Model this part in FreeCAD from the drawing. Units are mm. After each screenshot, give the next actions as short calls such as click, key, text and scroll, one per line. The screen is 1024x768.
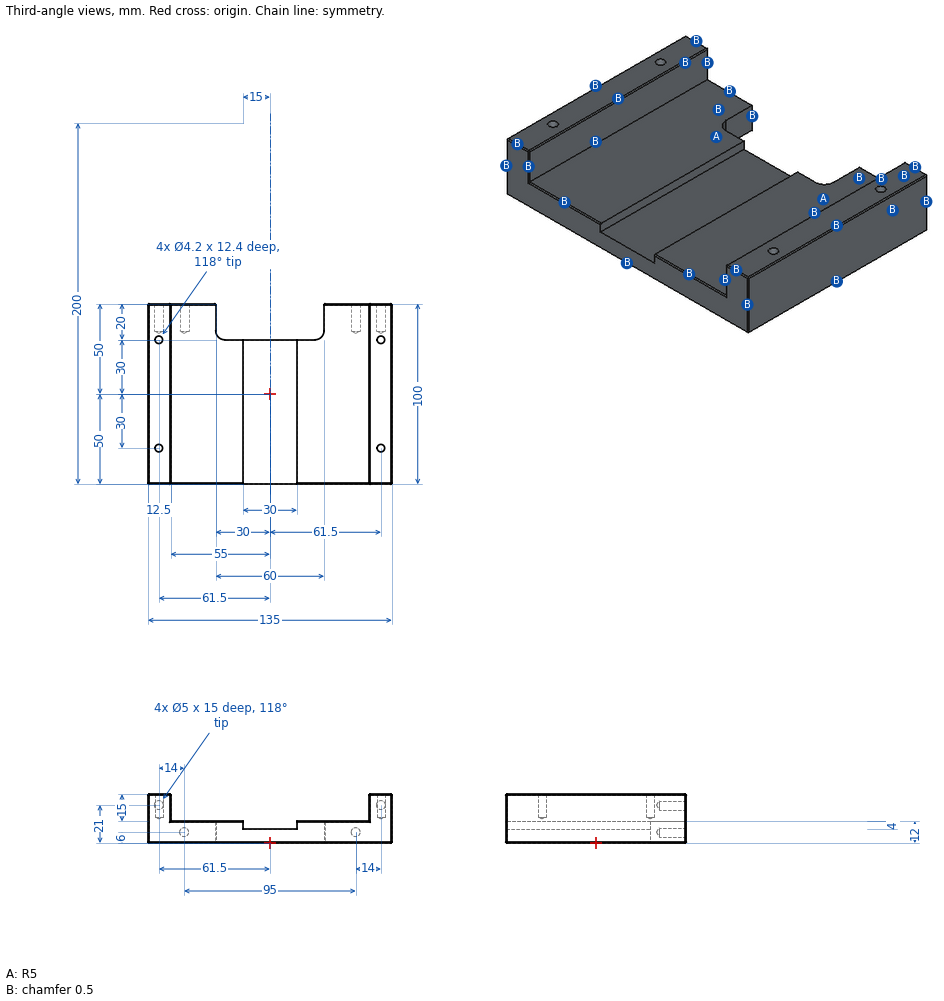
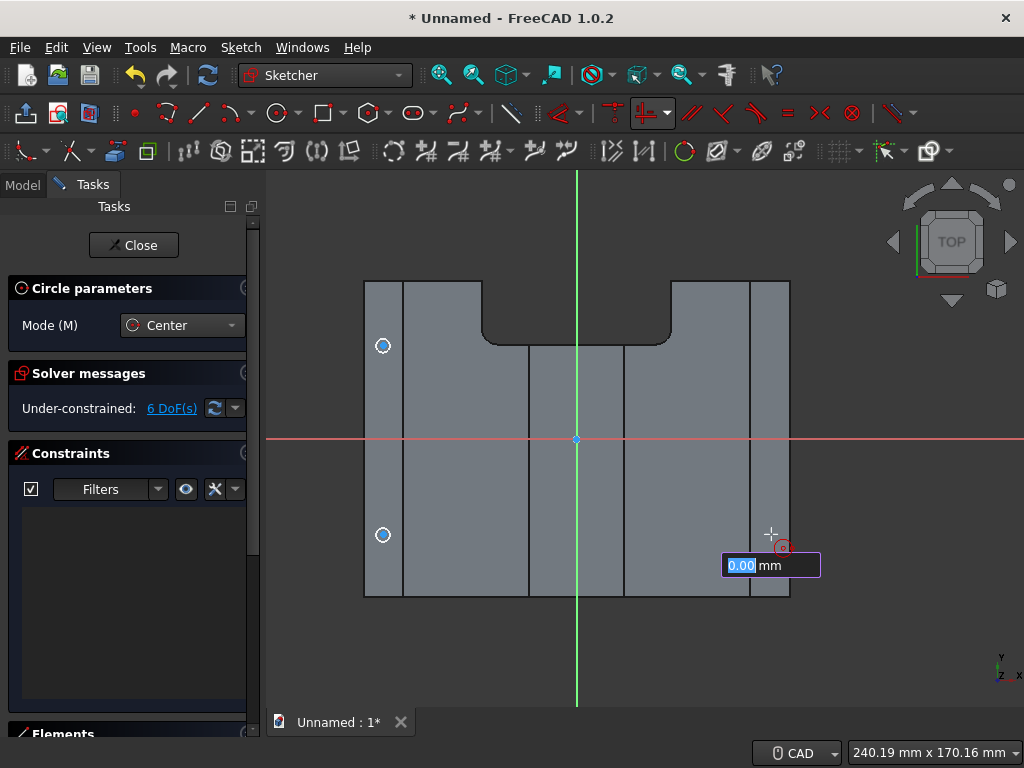
scroll(775, 529, up, 5)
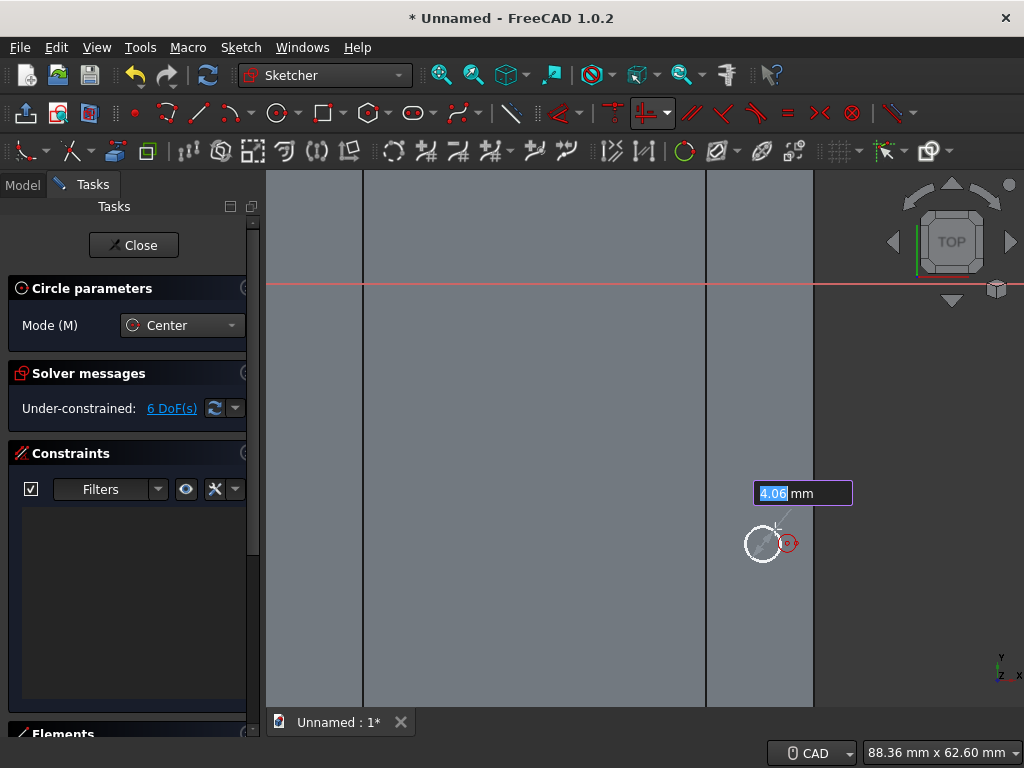
click(775, 528)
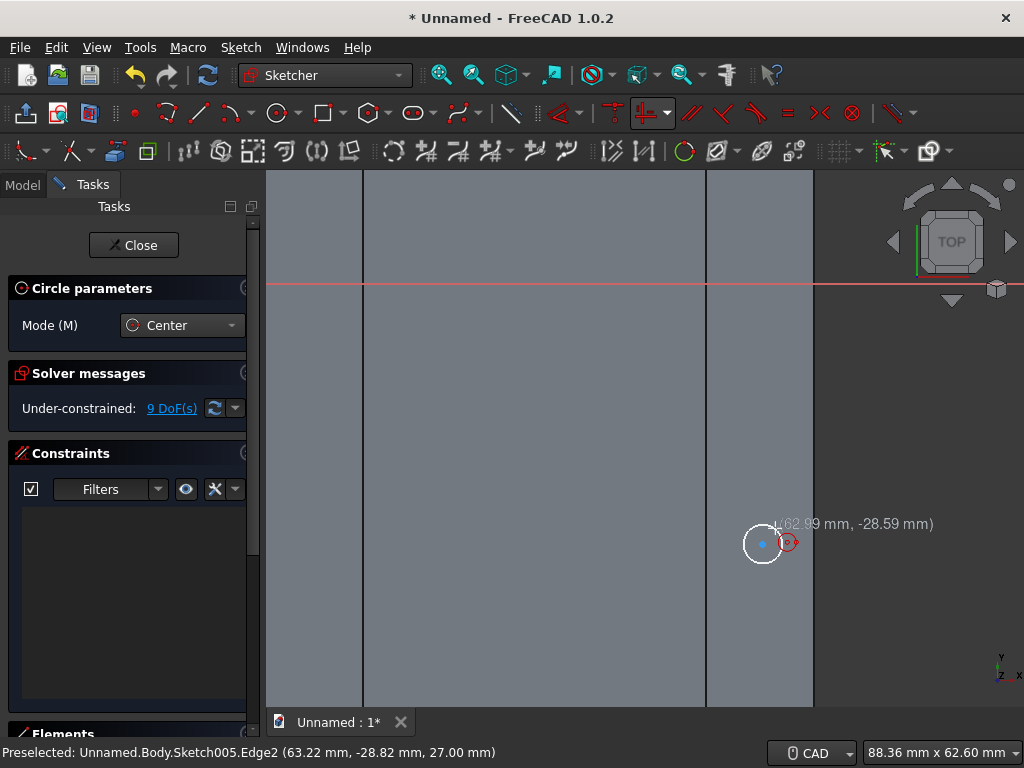
scroll(775, 529, down, 5)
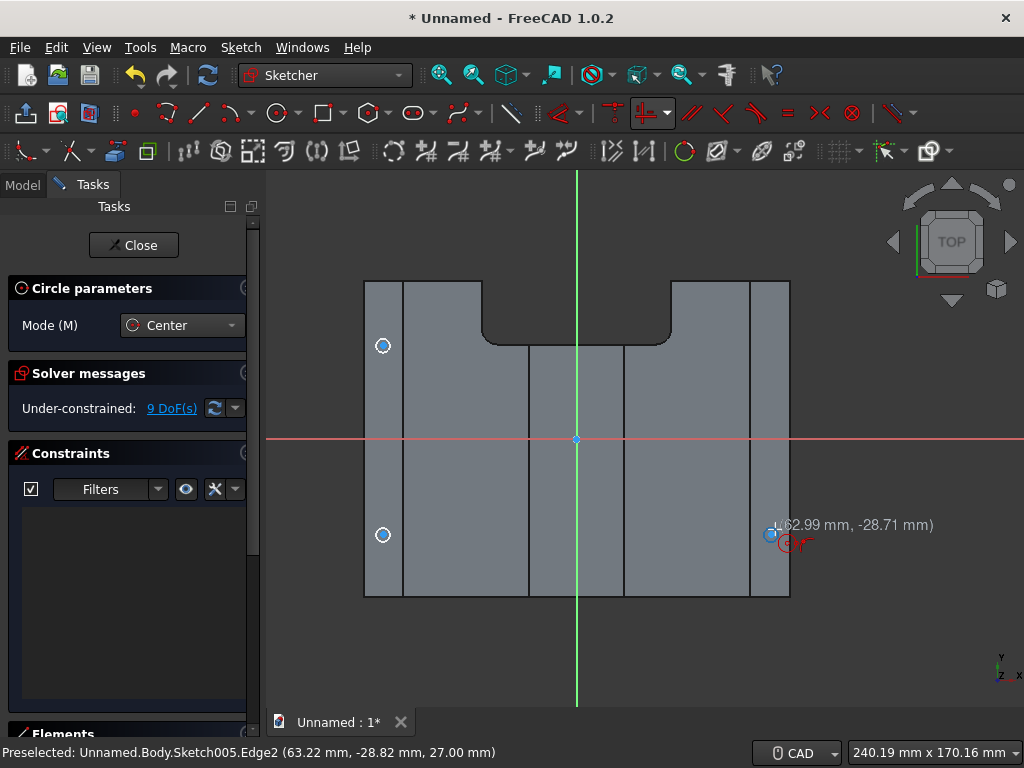
scroll(771, 345, up, 7)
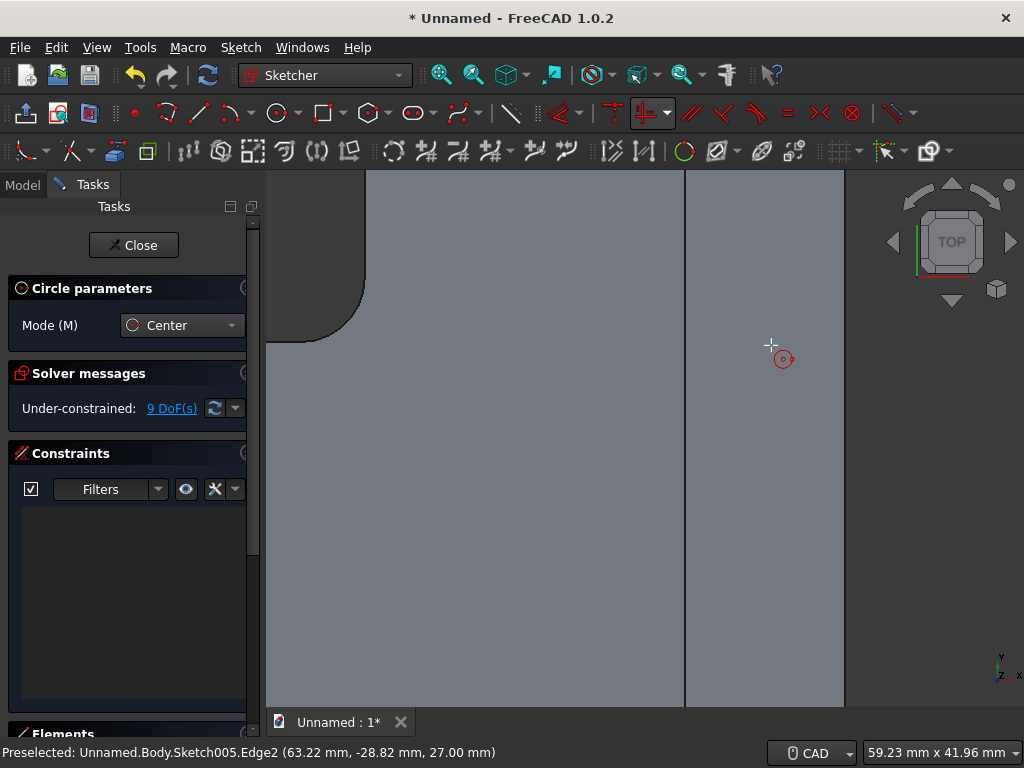
scroll(771, 344, down, 7)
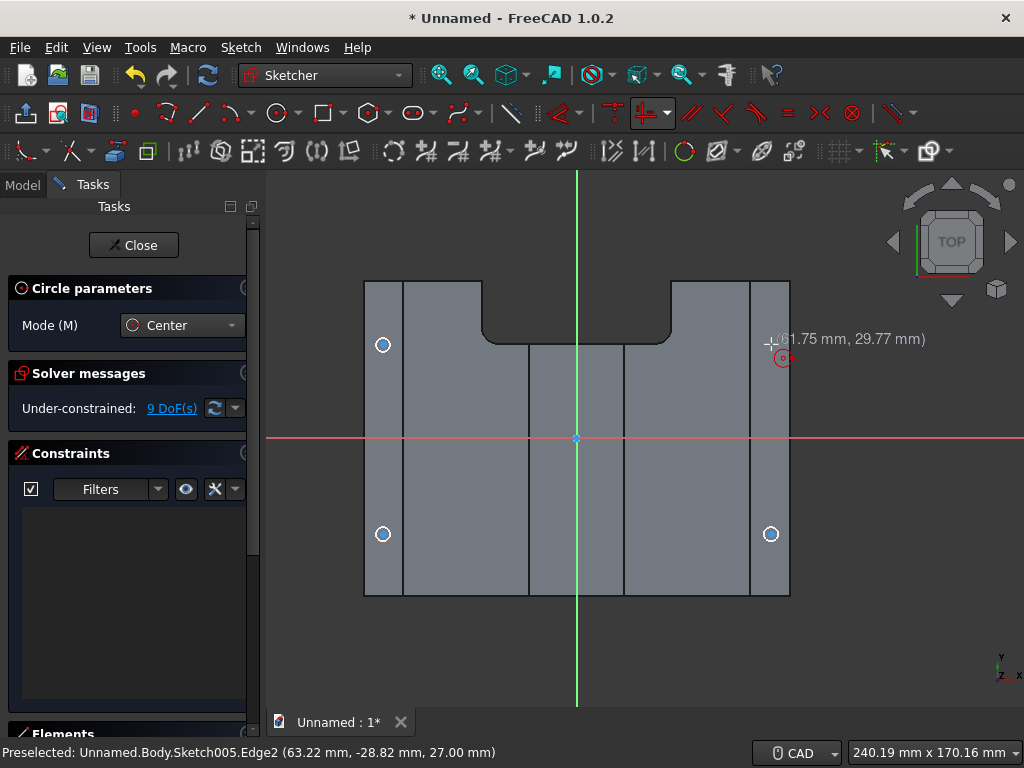
click(771, 344)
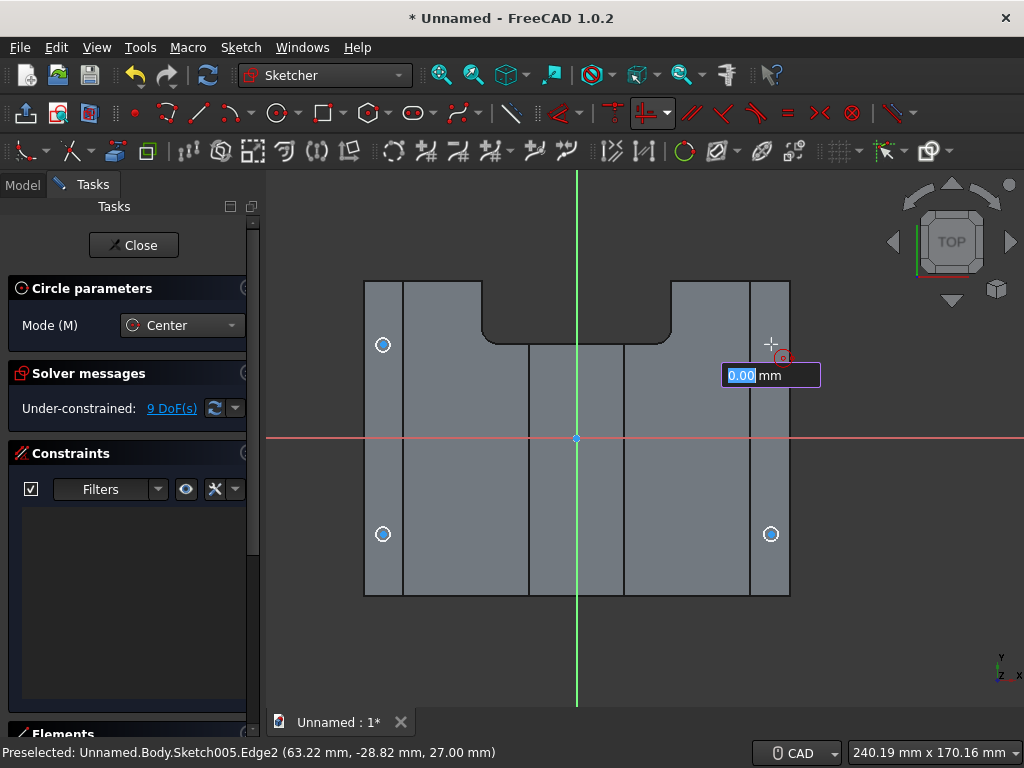
scroll(775, 339, up, 5)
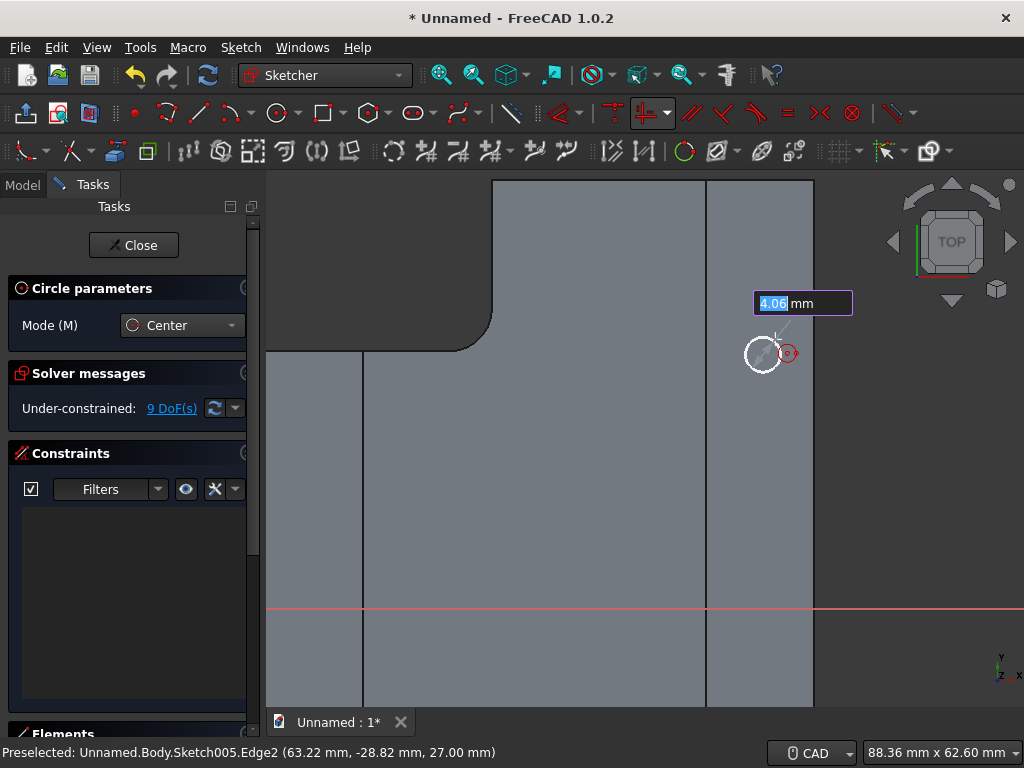
click(775, 339)
key(Escape)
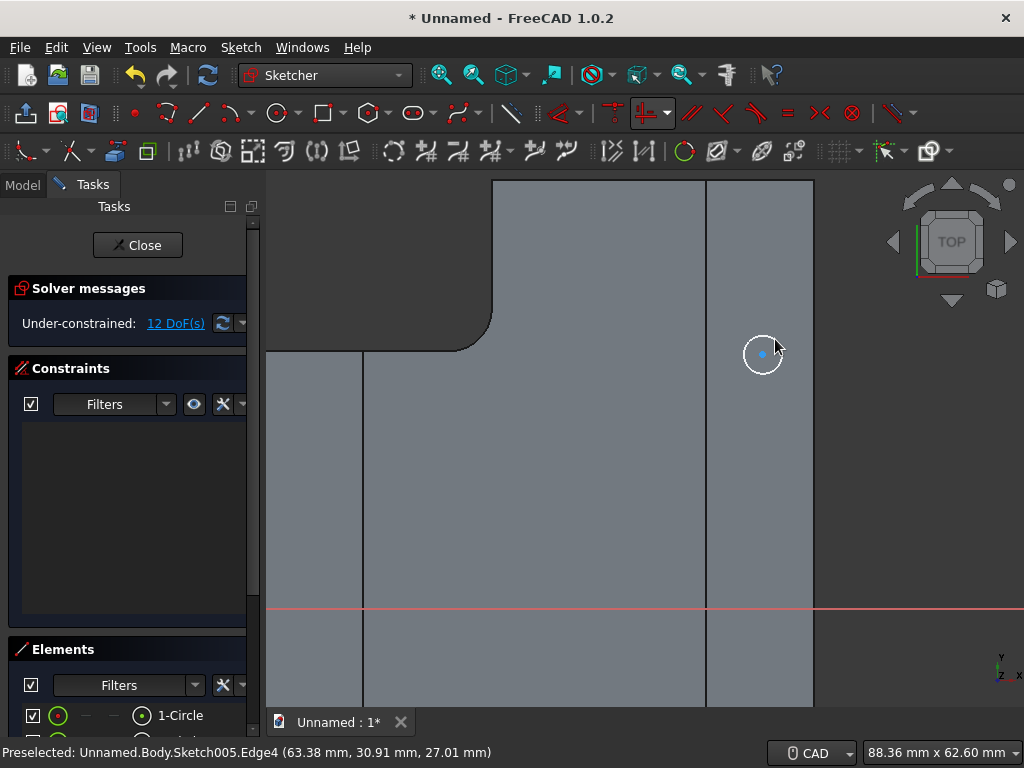
scroll(775, 339, down, 5)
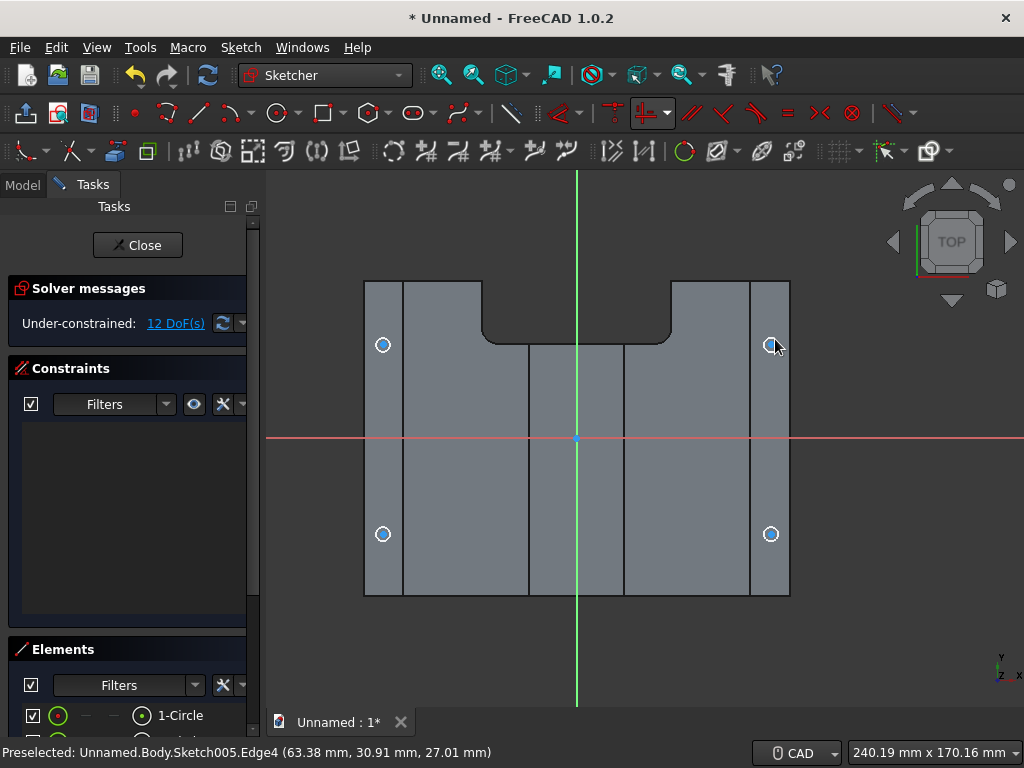
scroll(388, 340, up, 4)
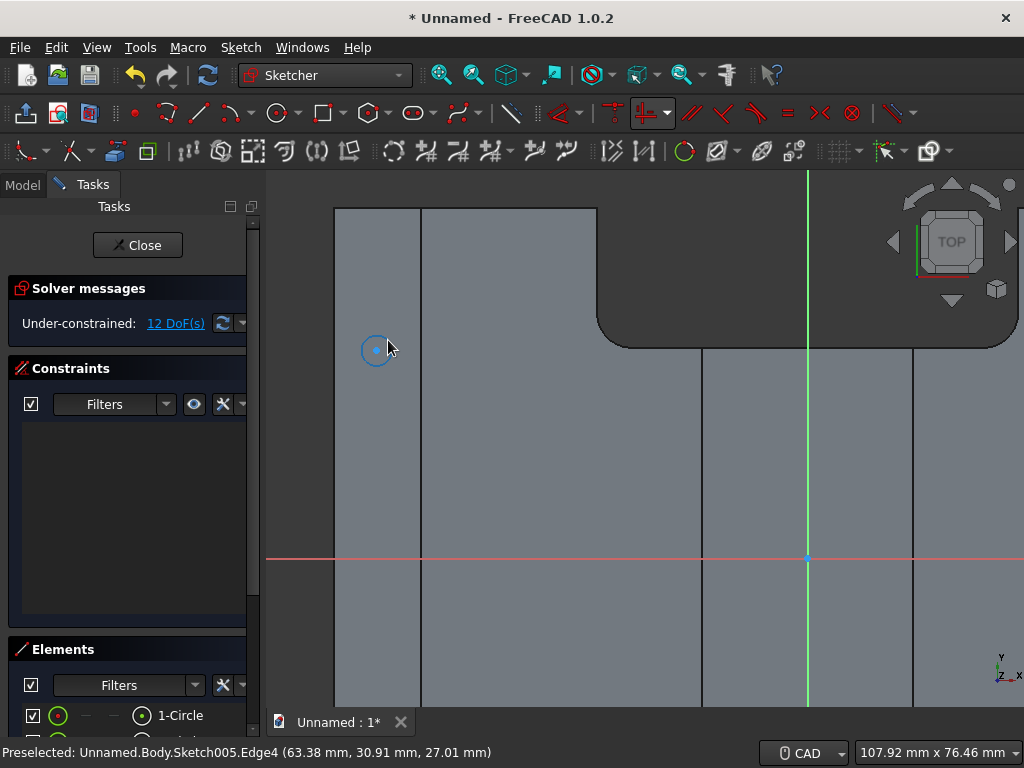
click(387, 340)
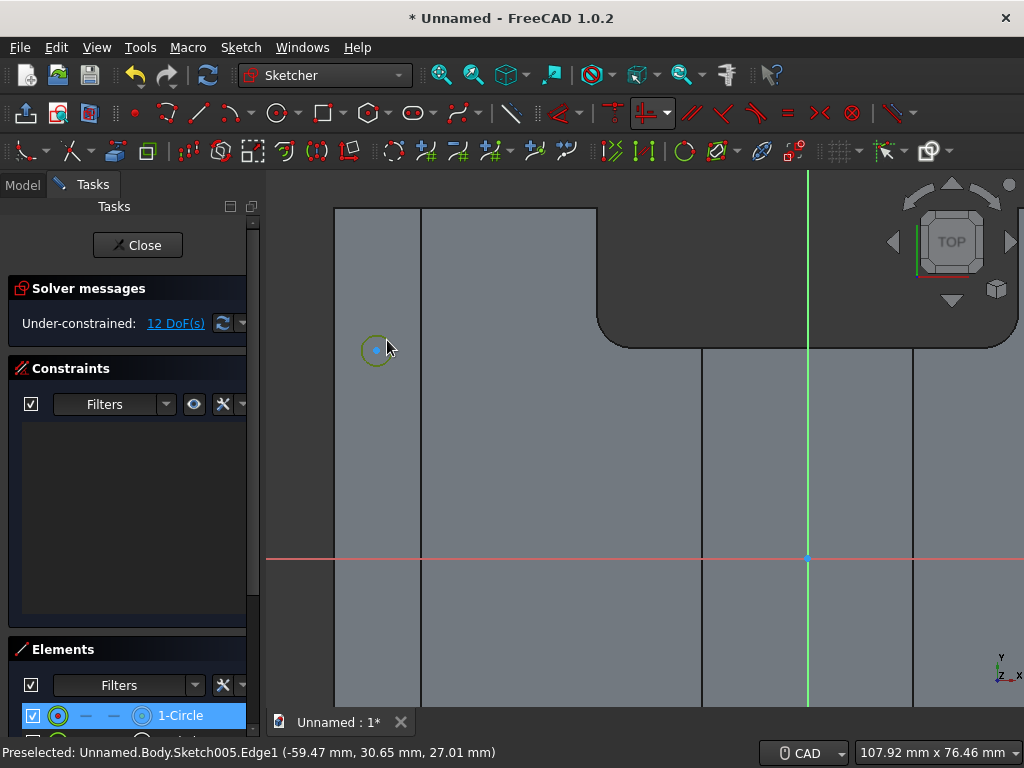
scroll(388, 340, down, 4)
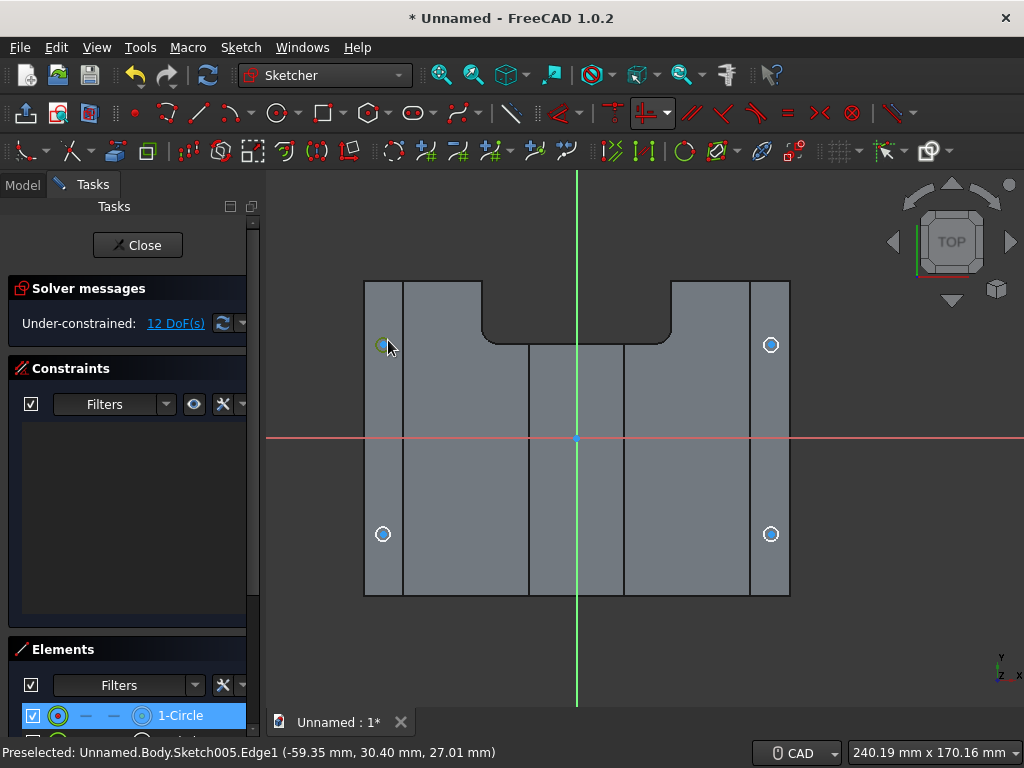
scroll(388, 529, up, 4)